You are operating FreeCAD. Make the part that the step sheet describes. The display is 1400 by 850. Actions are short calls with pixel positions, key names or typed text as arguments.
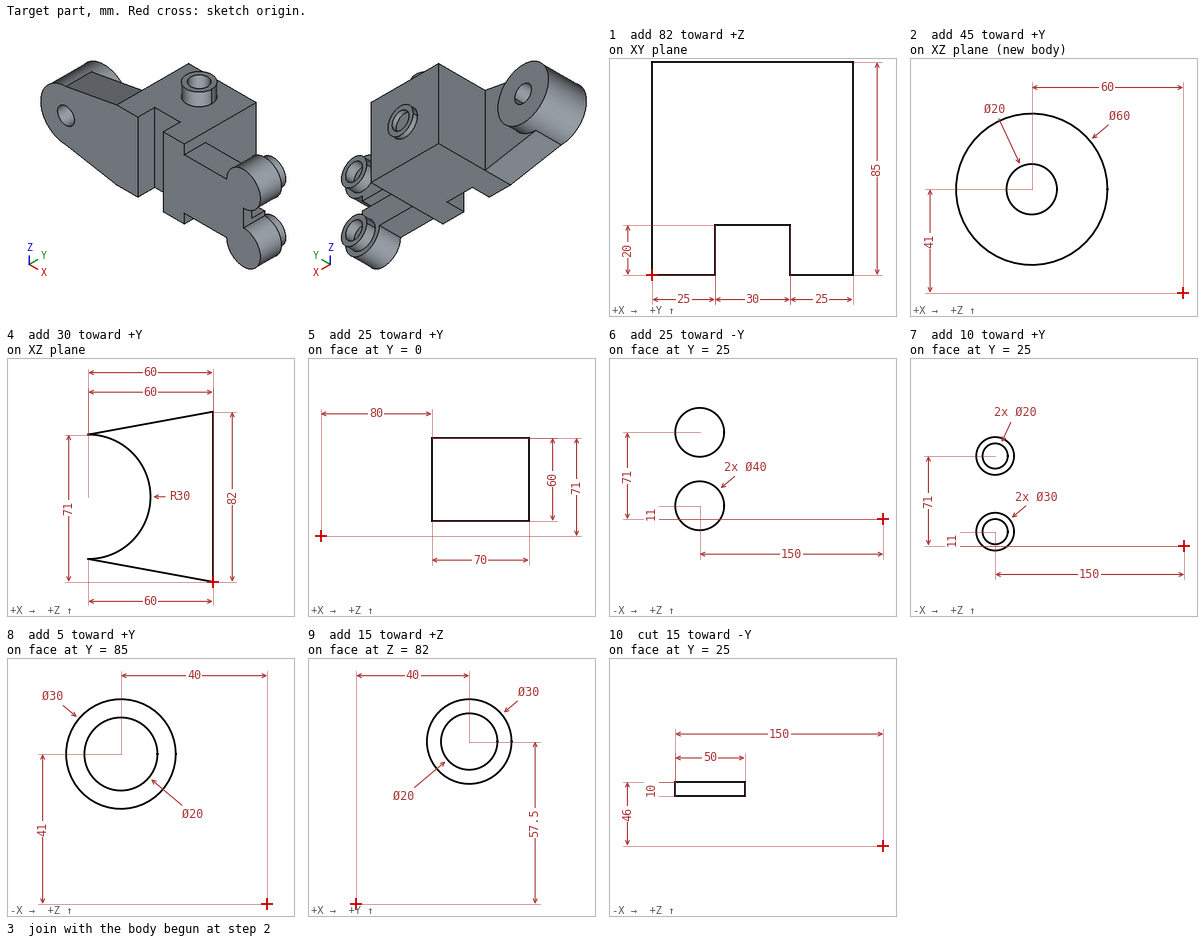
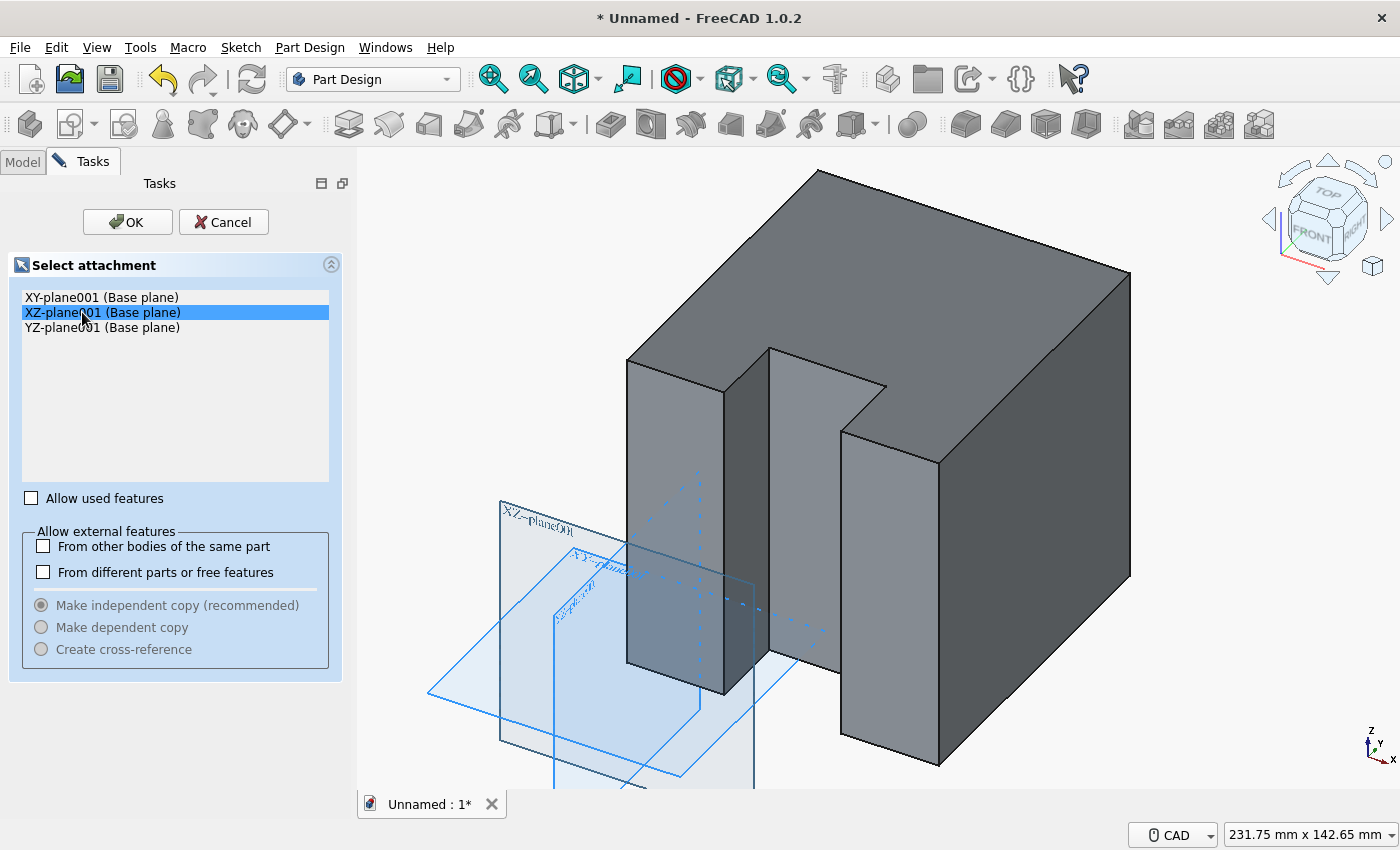
click(128, 222)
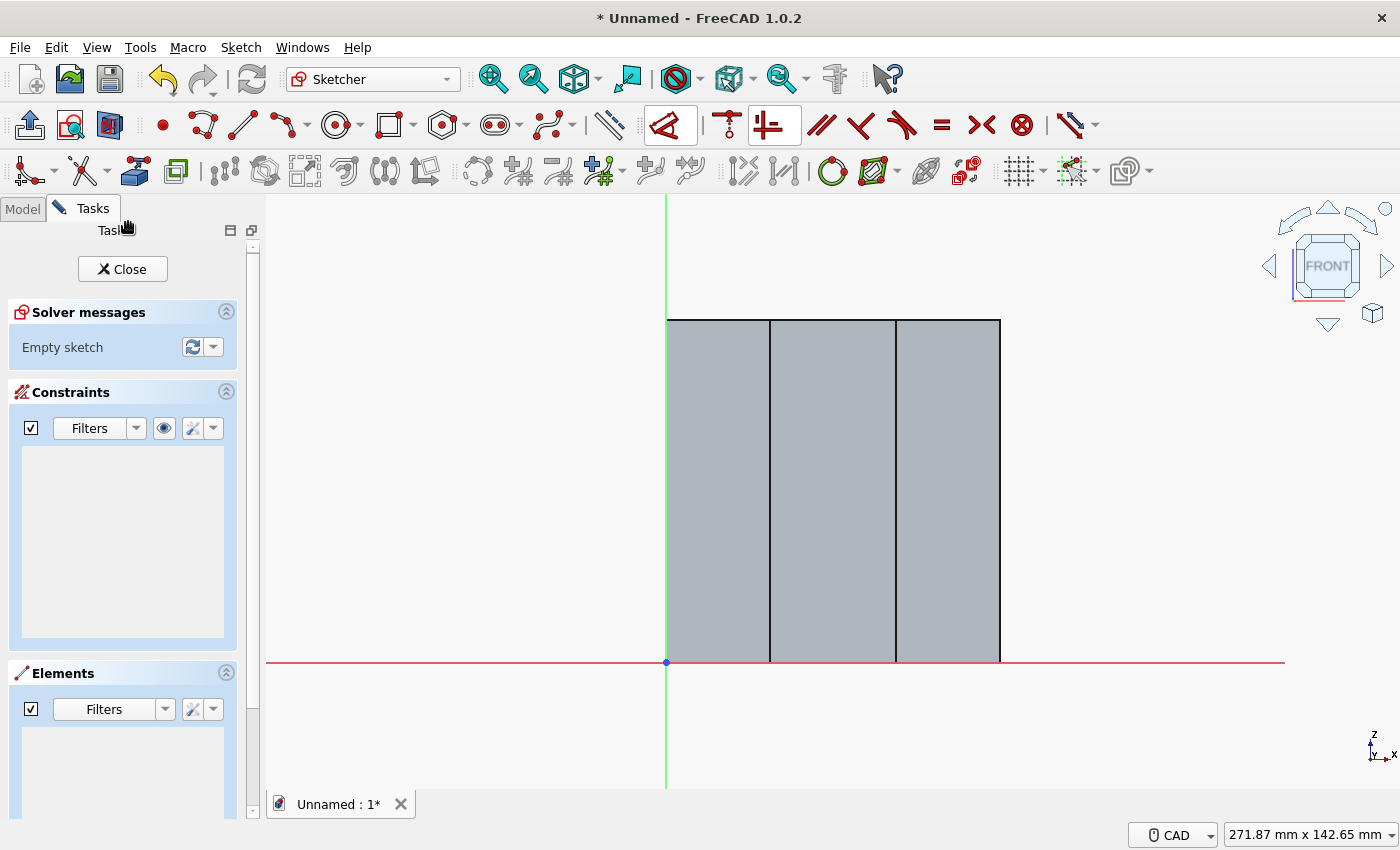
scroll(1235, 388, down, 1)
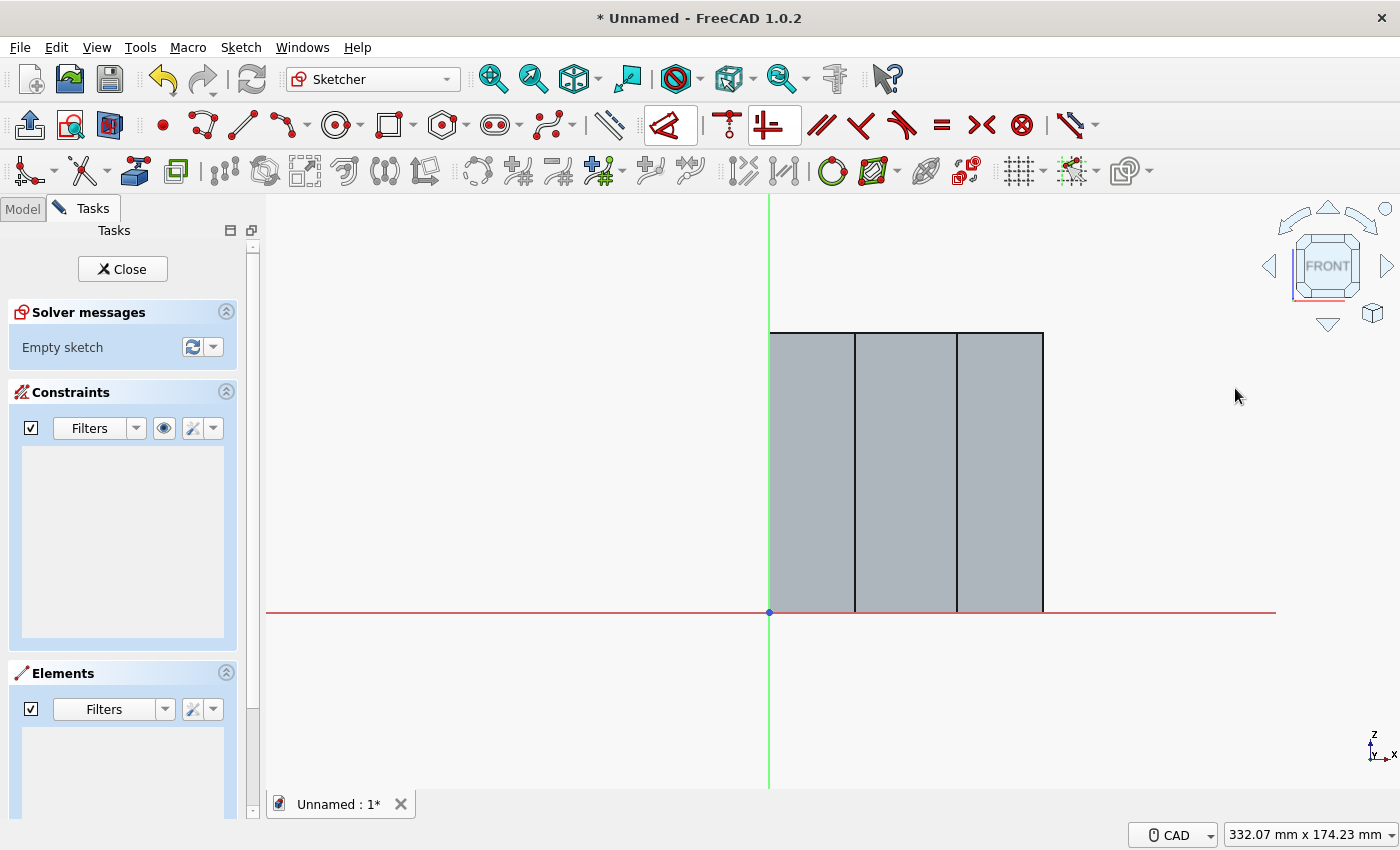
scroll(313, 492, up, 2)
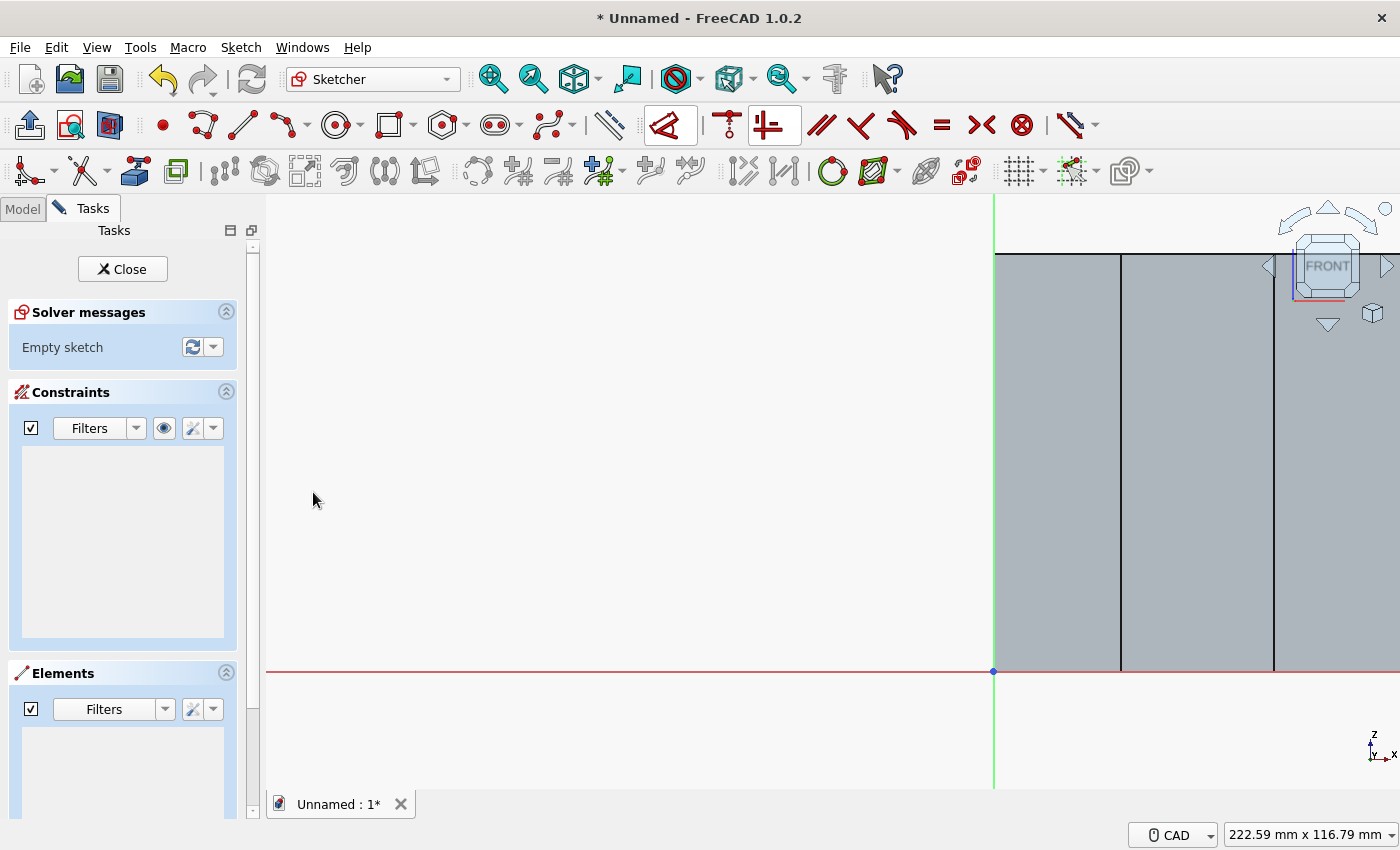
key(g)
key(c)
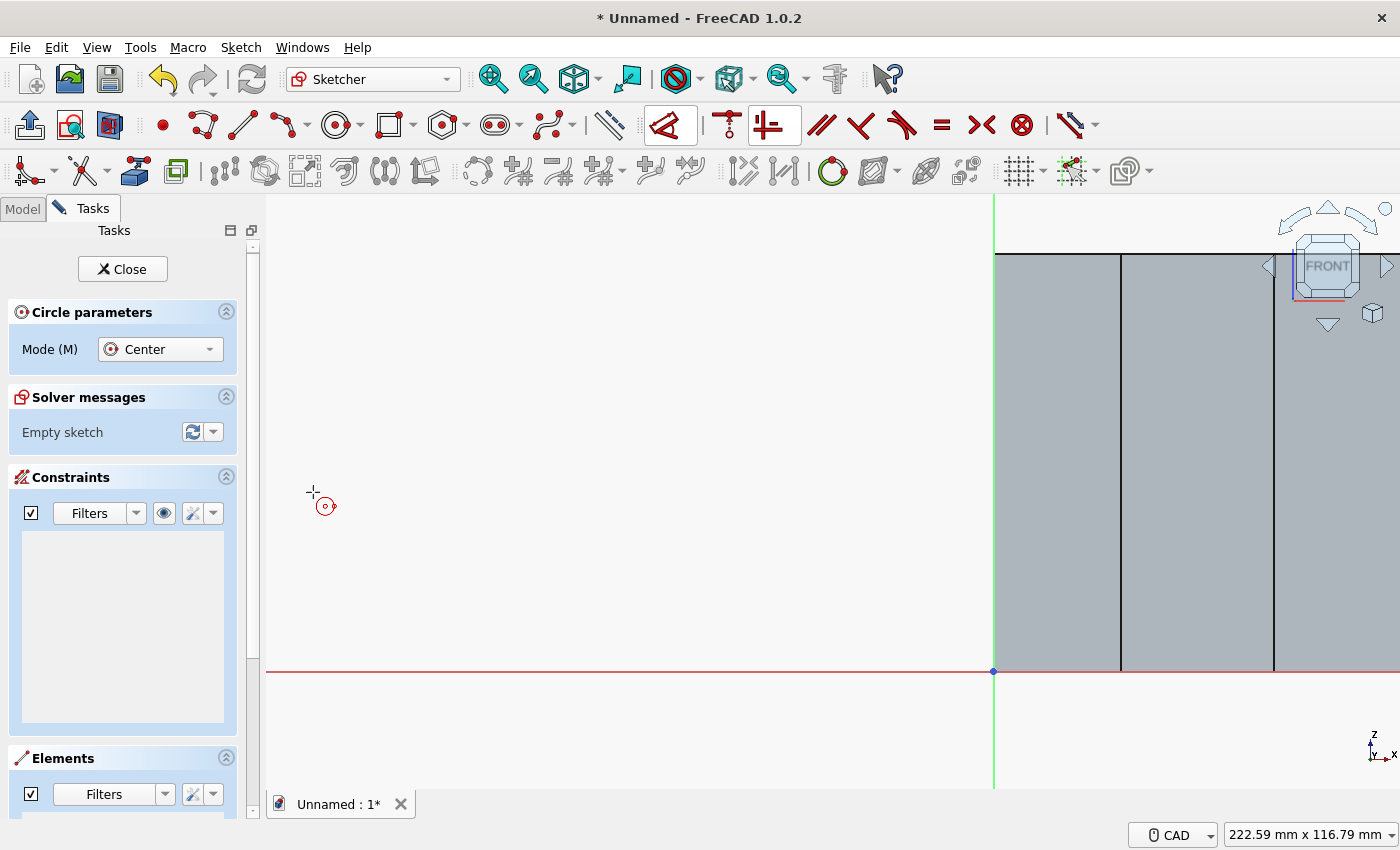
click(688, 463)
click(796, 355)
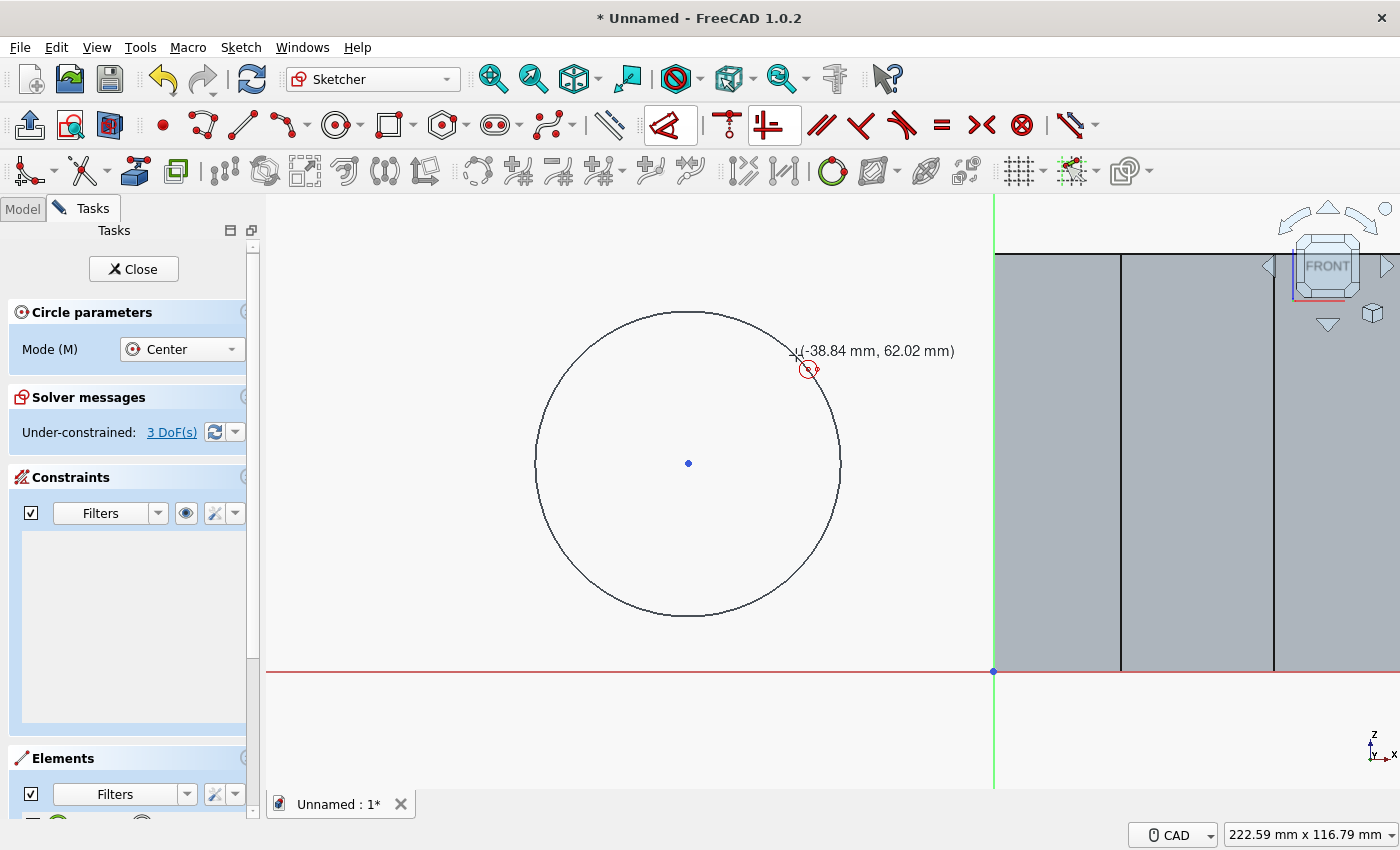
click(688, 464)
click(724, 427)
key(Escape)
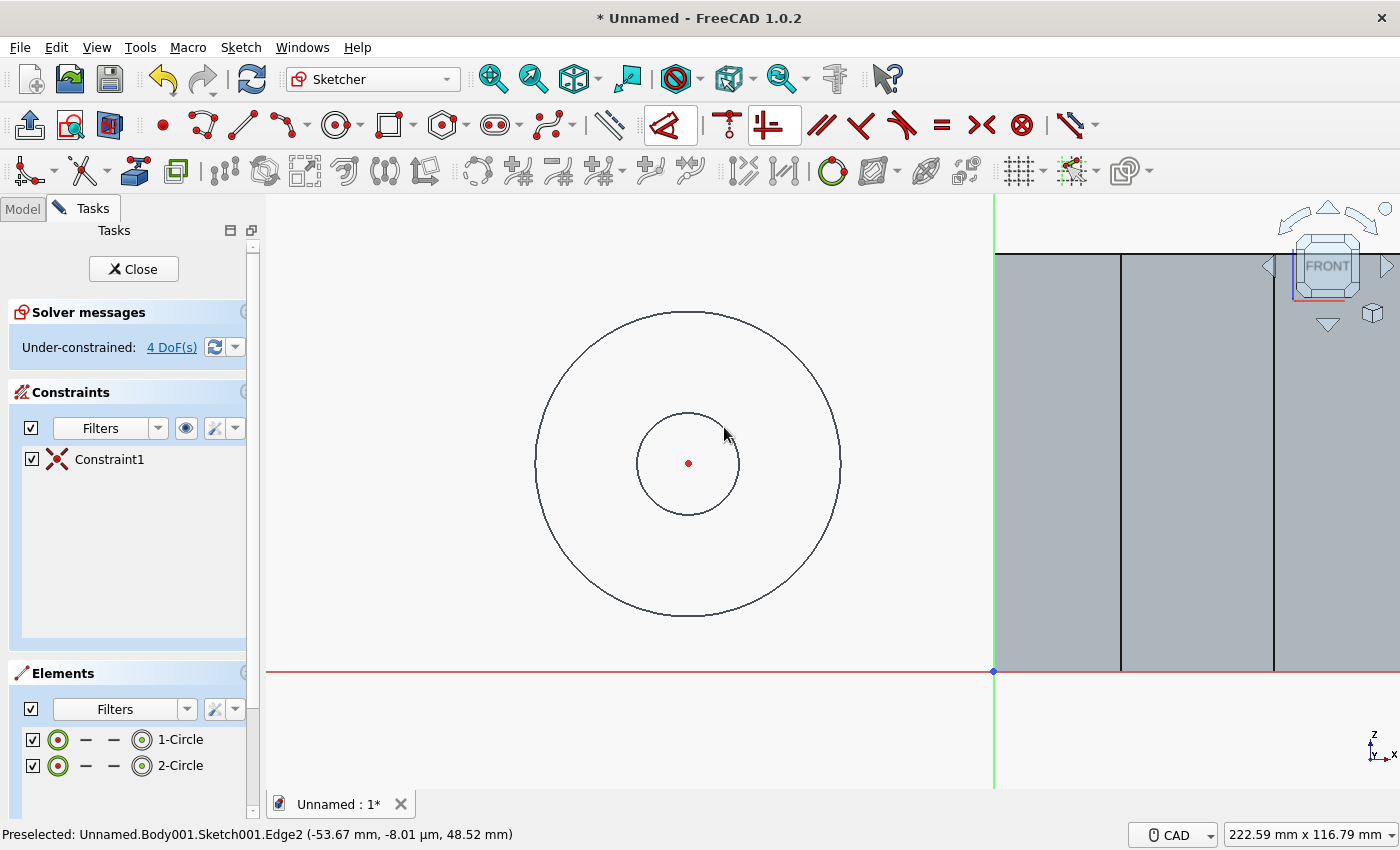
click(796, 356)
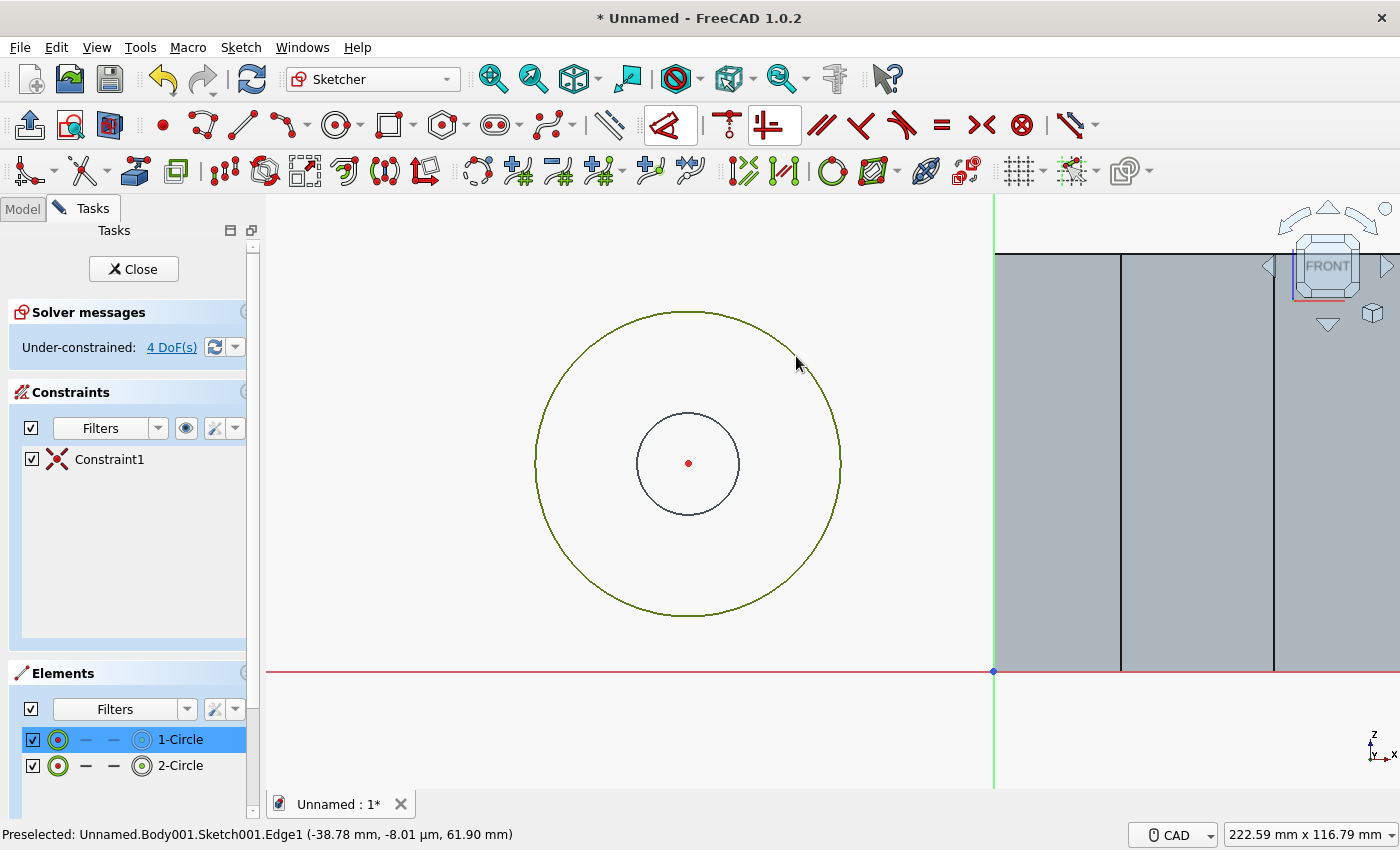
key(k)
key(o)